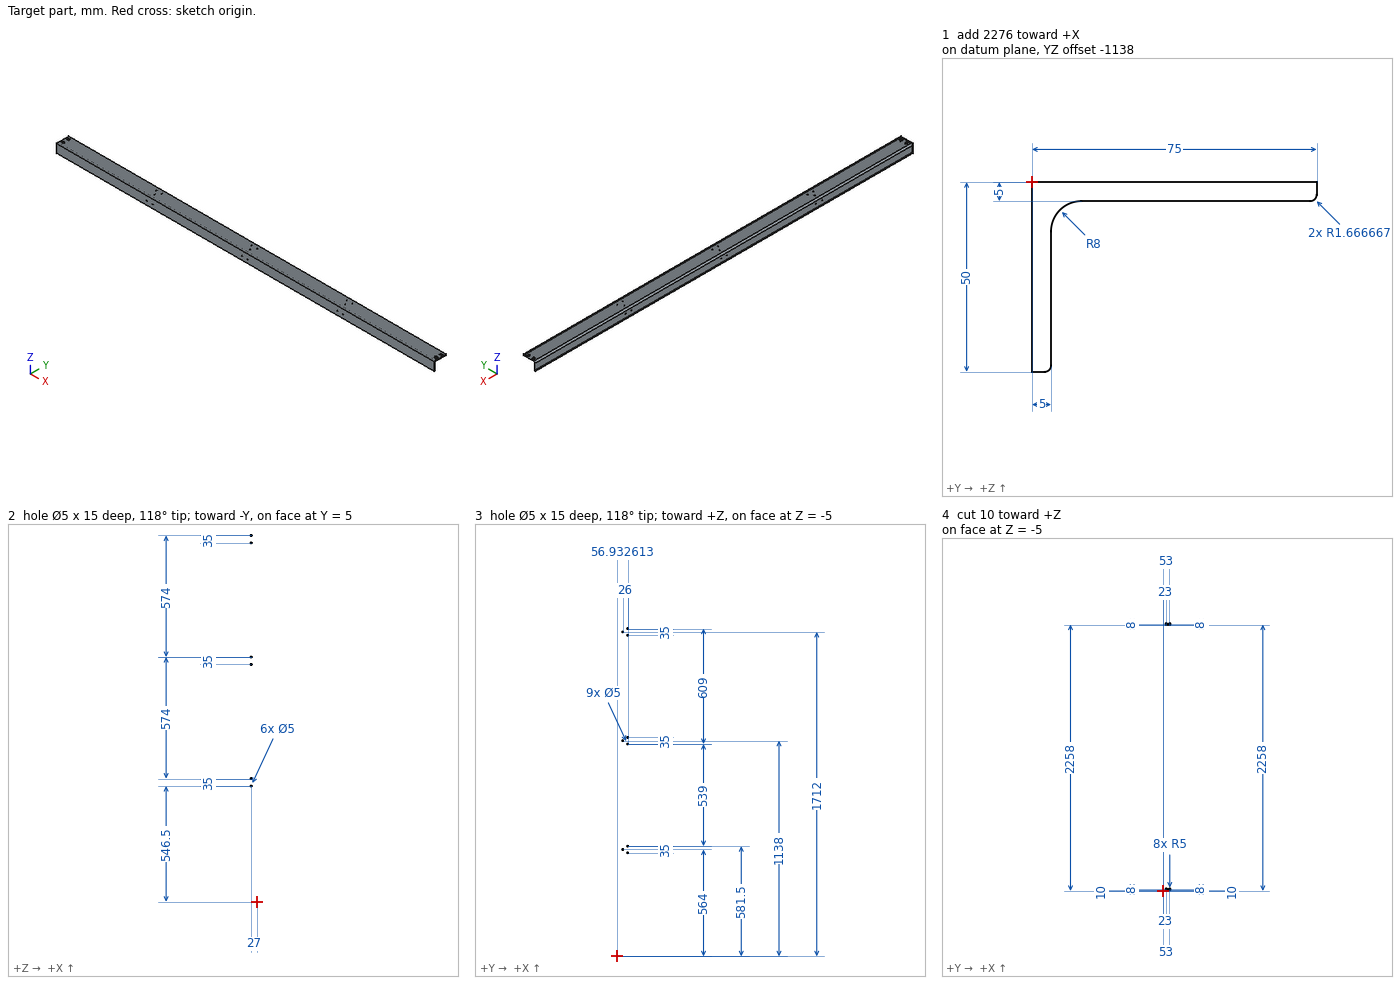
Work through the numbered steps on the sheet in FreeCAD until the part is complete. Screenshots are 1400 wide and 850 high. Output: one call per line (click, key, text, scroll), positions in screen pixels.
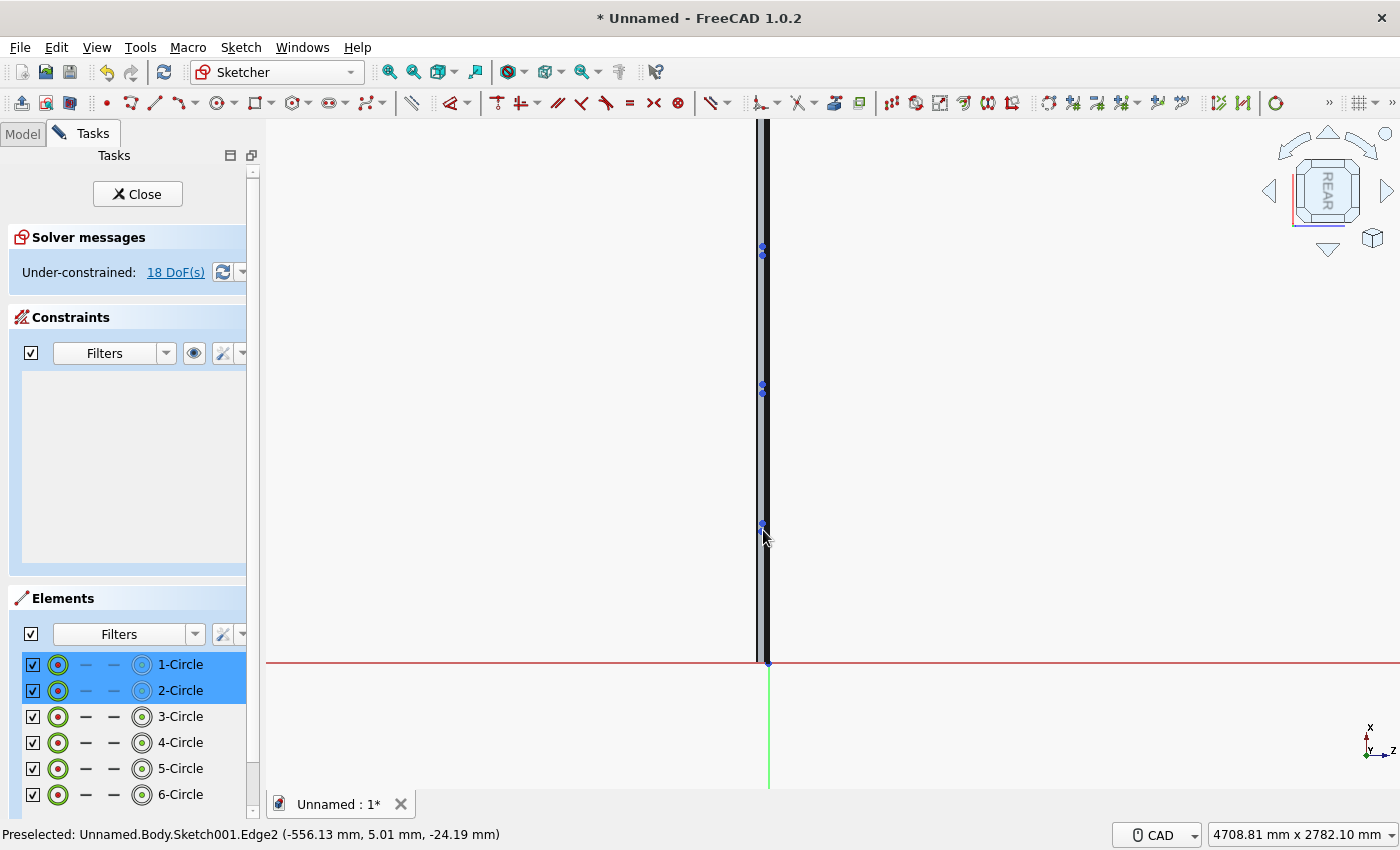
scroll(763, 384, up, 14)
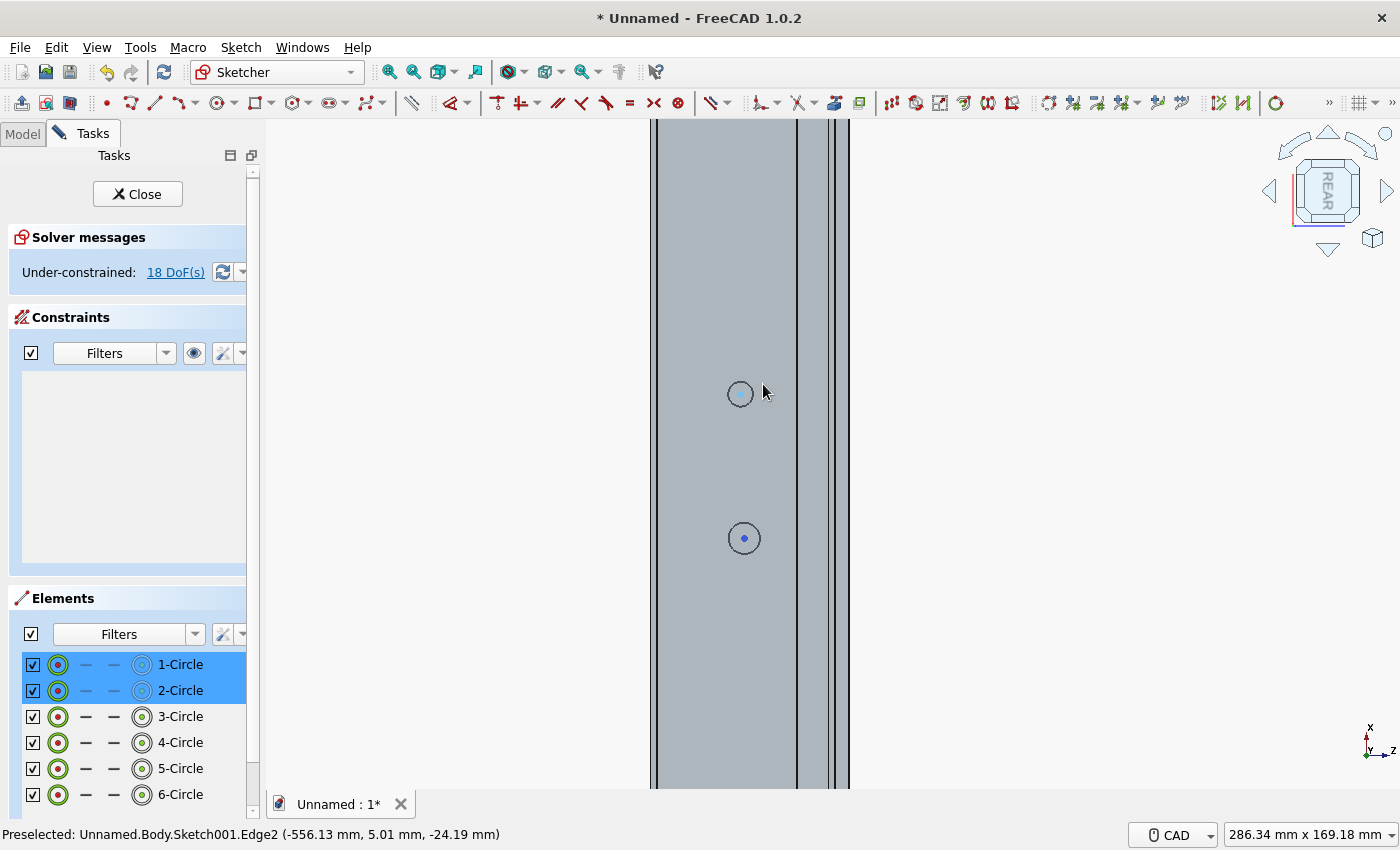
click(749, 385)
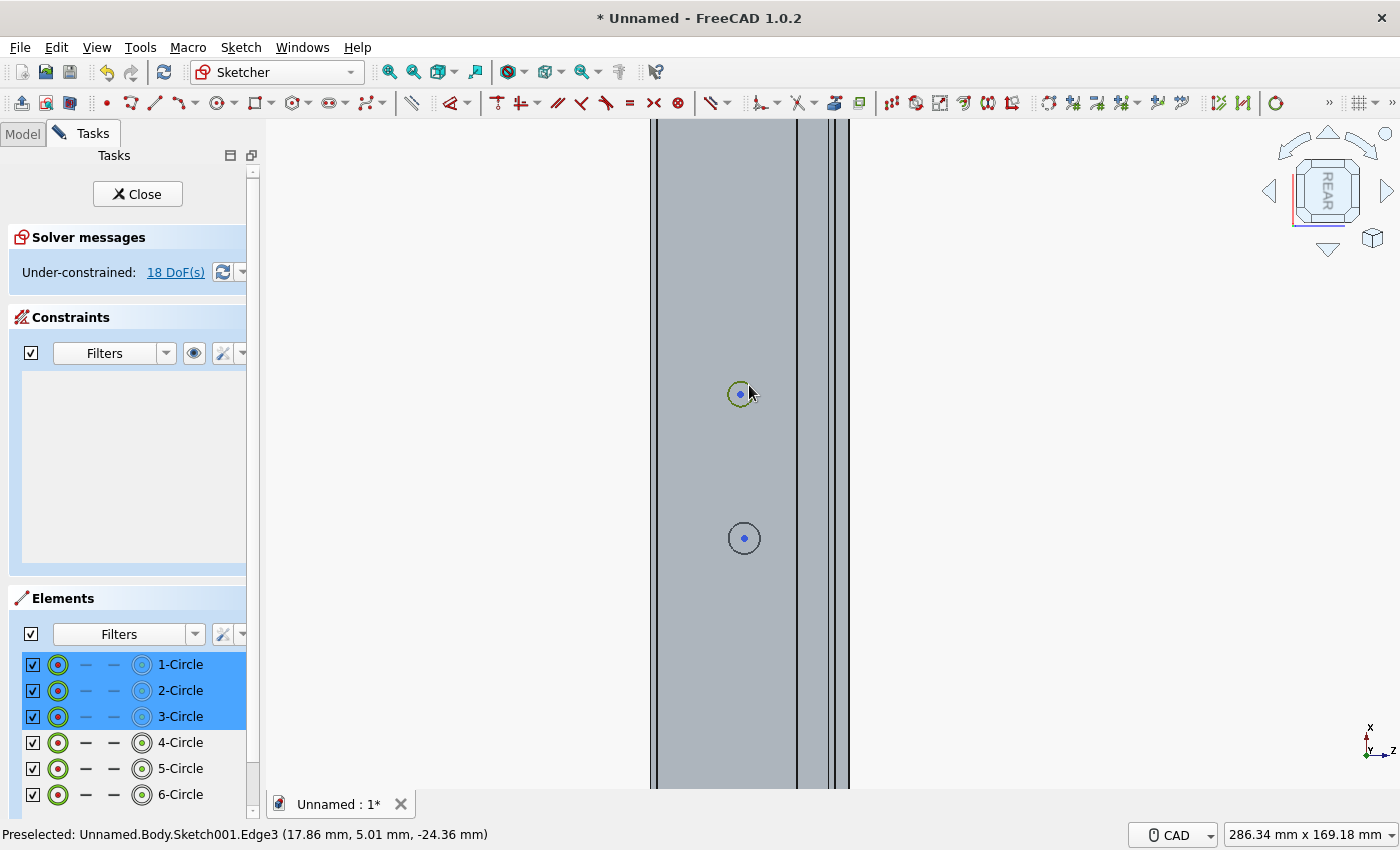
click(755, 527)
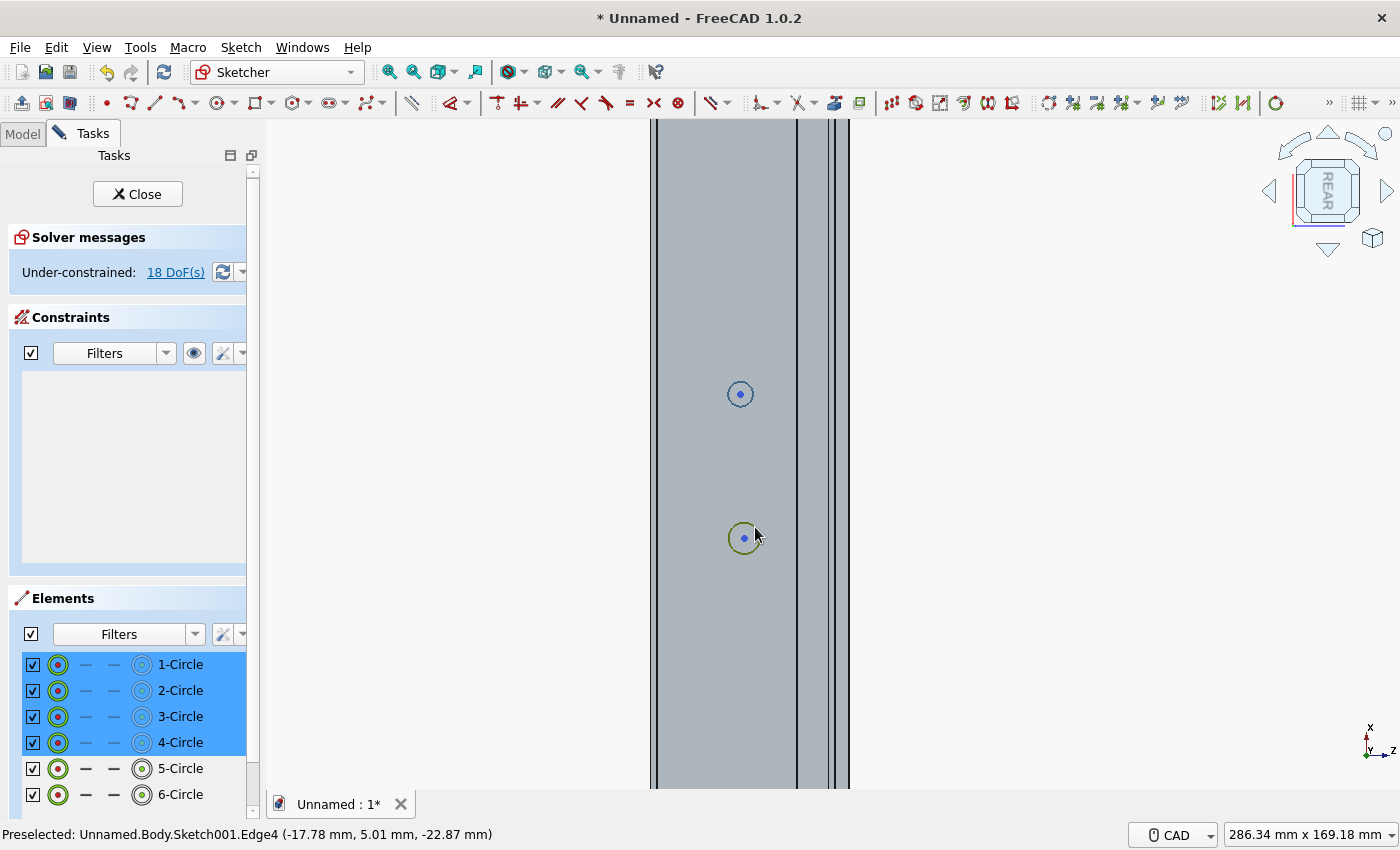
scroll(763, 384, down, 14)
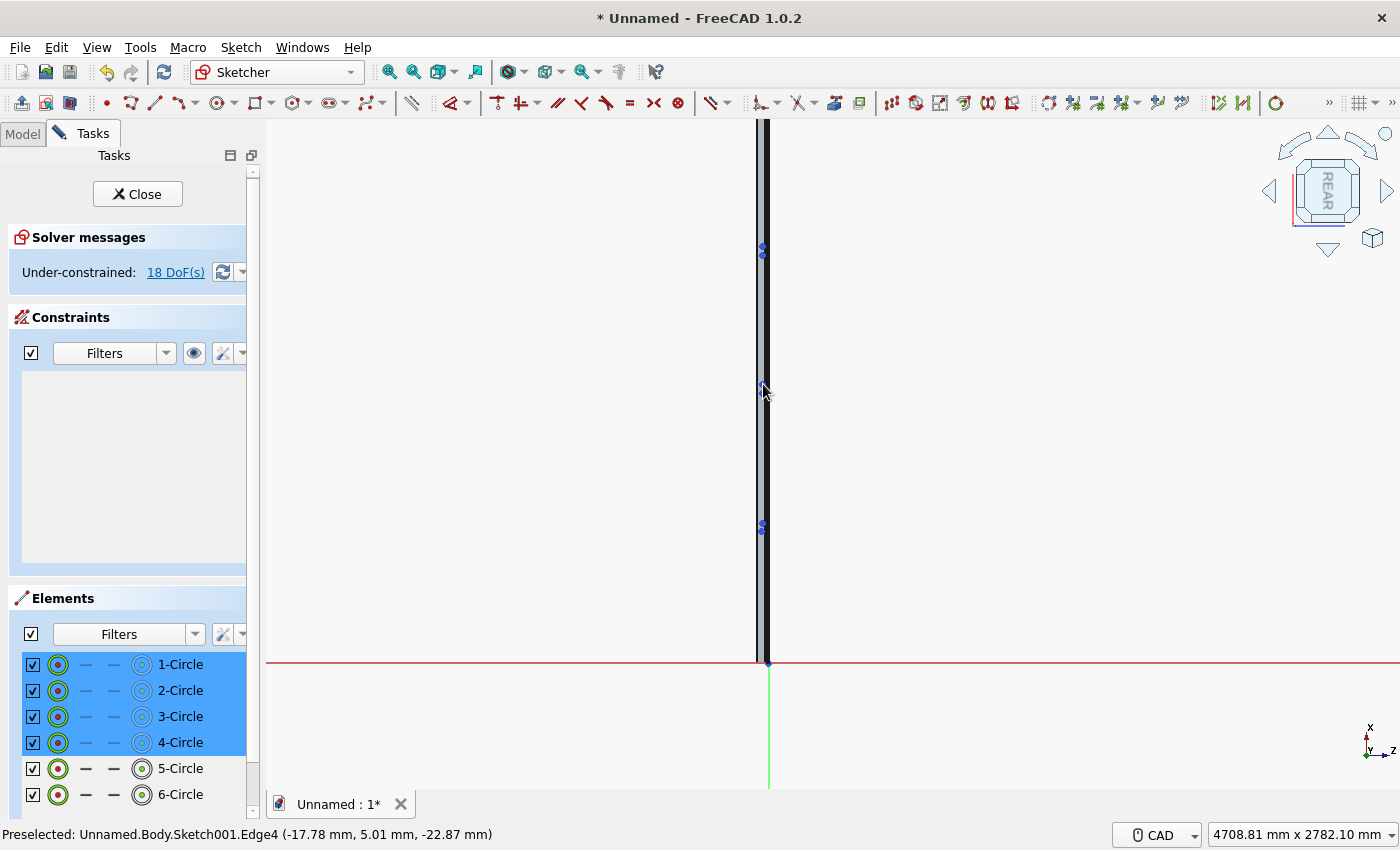
scroll(763, 246, up, 14)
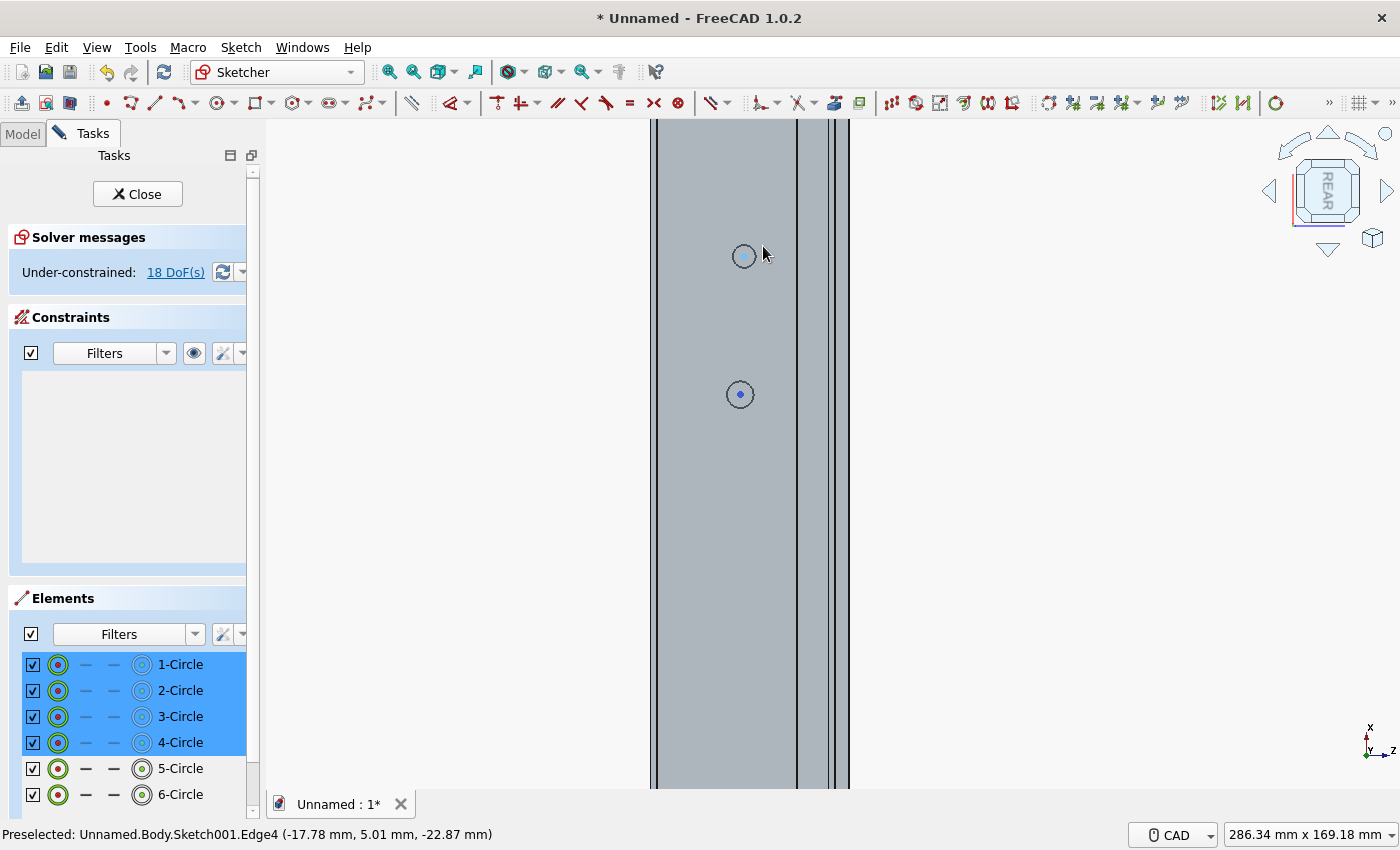
click(752, 248)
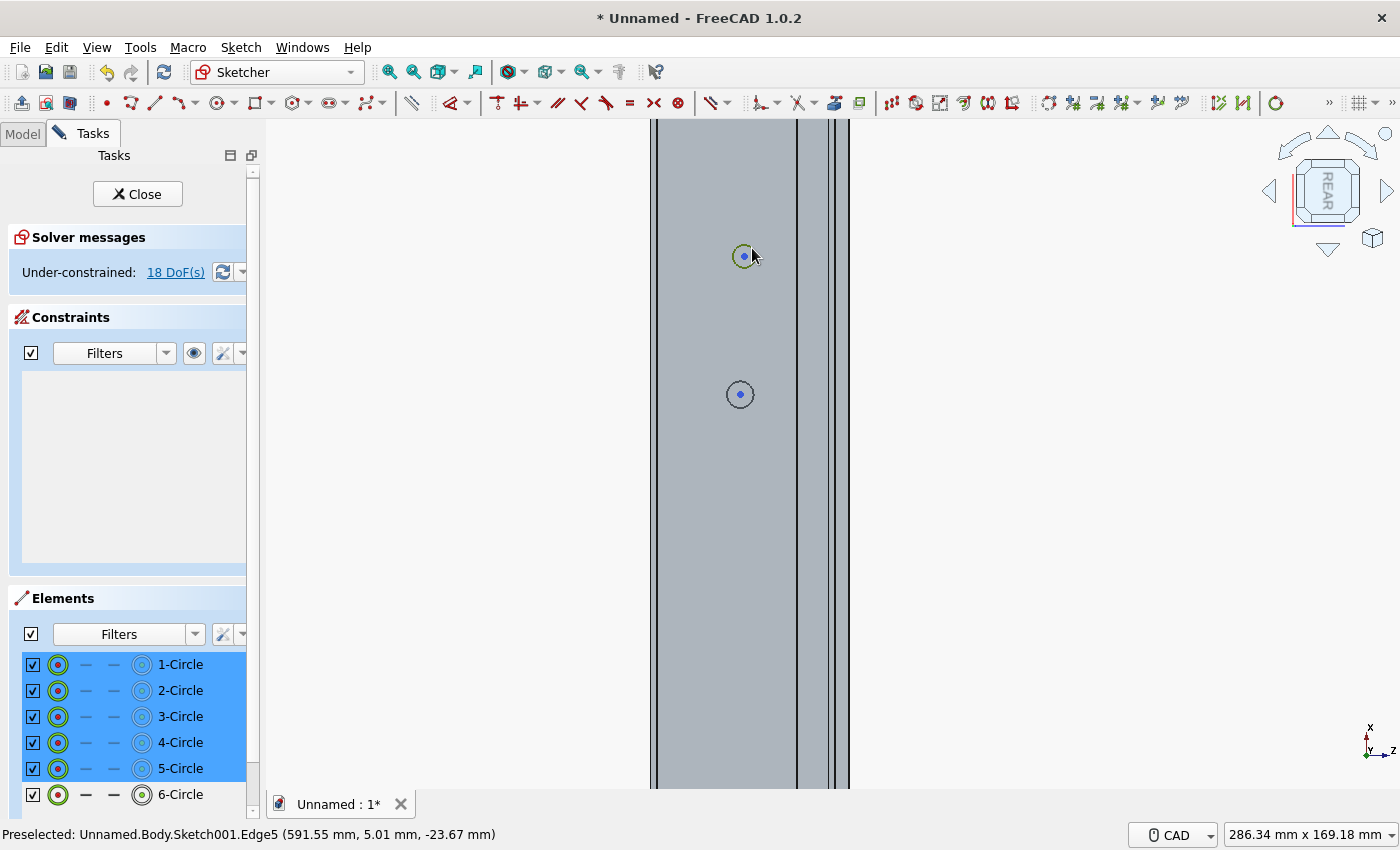
click(750, 385)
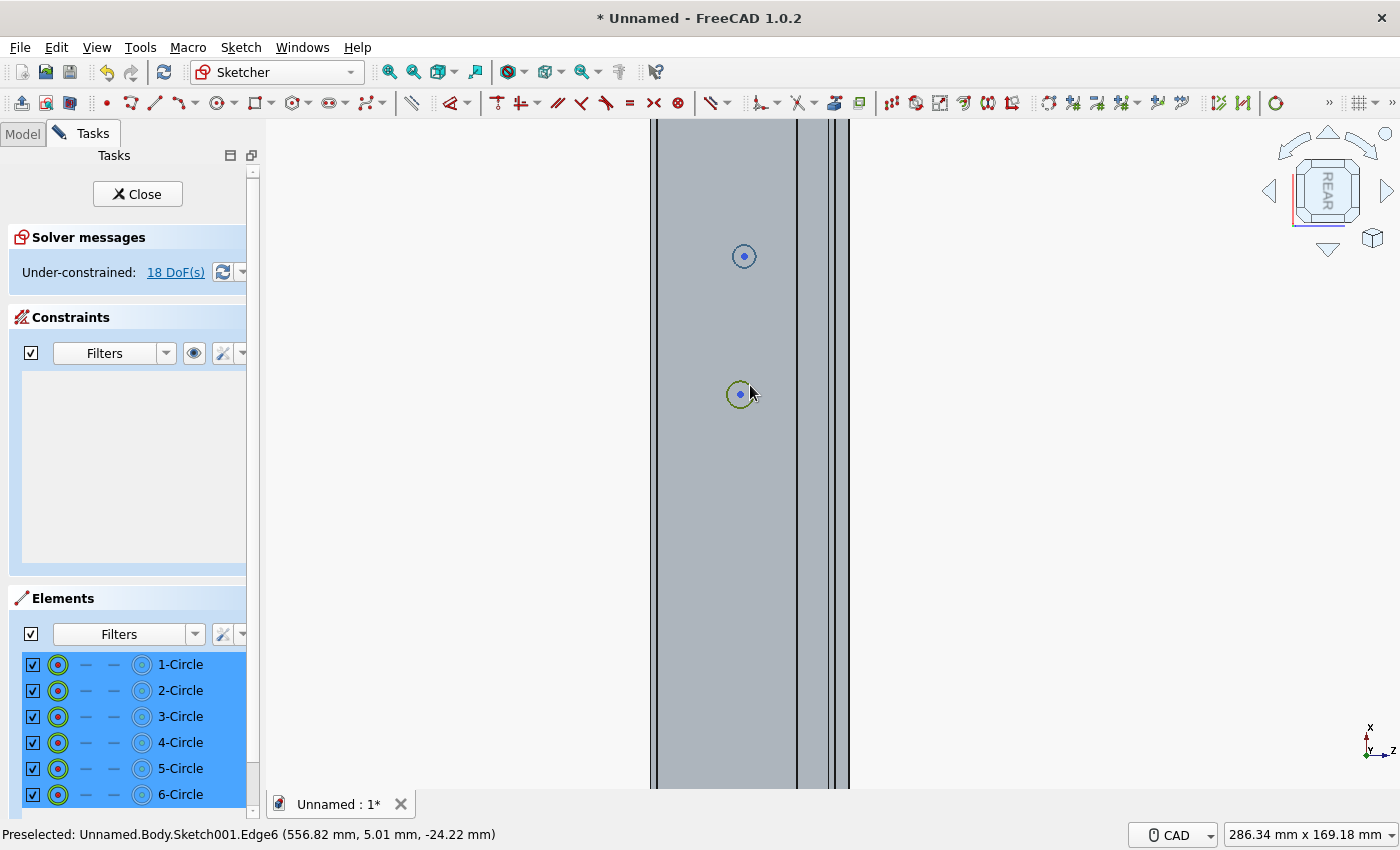
click(630, 104)